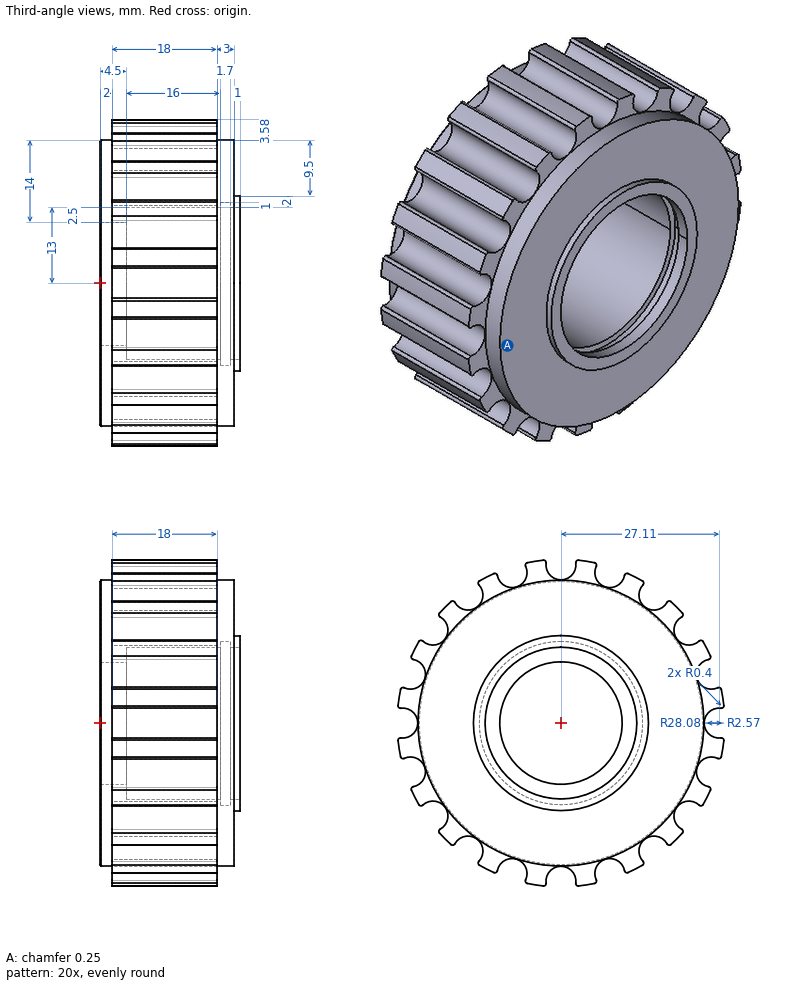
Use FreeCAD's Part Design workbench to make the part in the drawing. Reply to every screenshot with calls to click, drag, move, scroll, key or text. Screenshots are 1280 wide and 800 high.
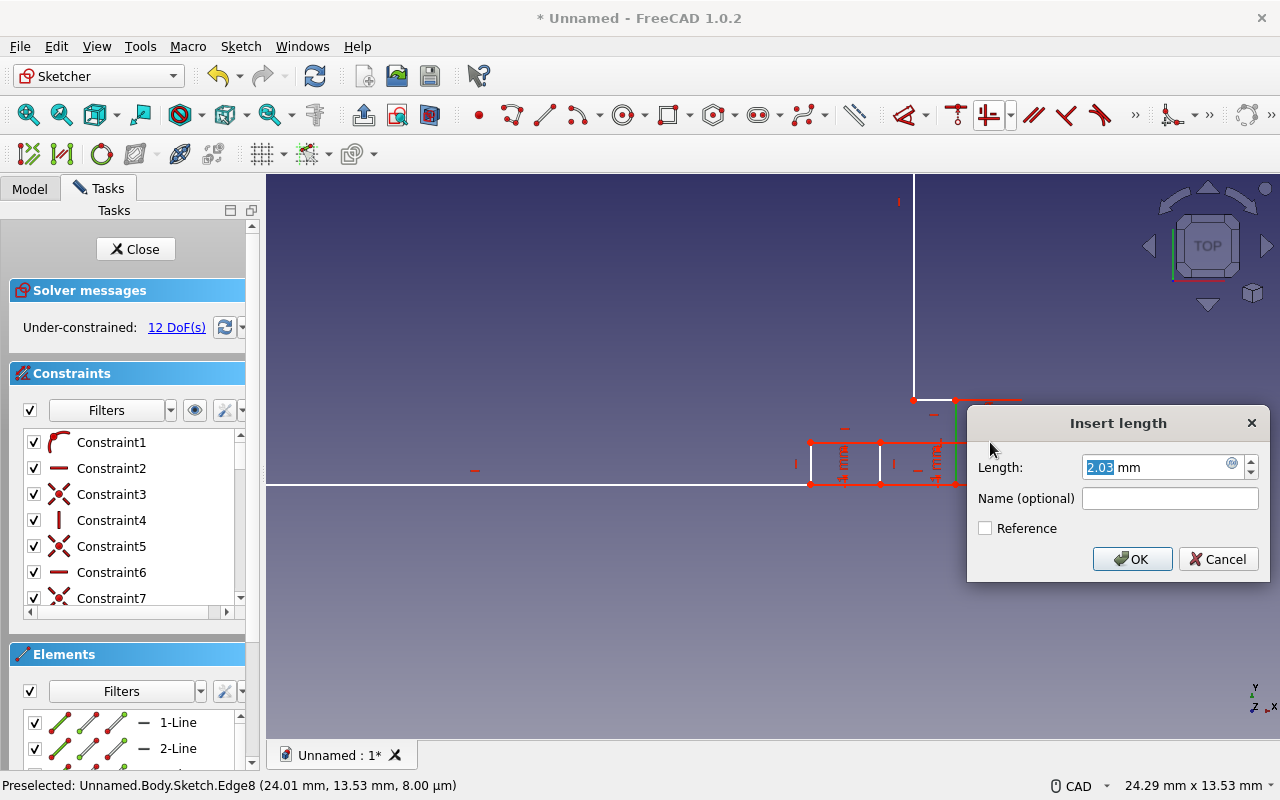
text(2)
key(Return)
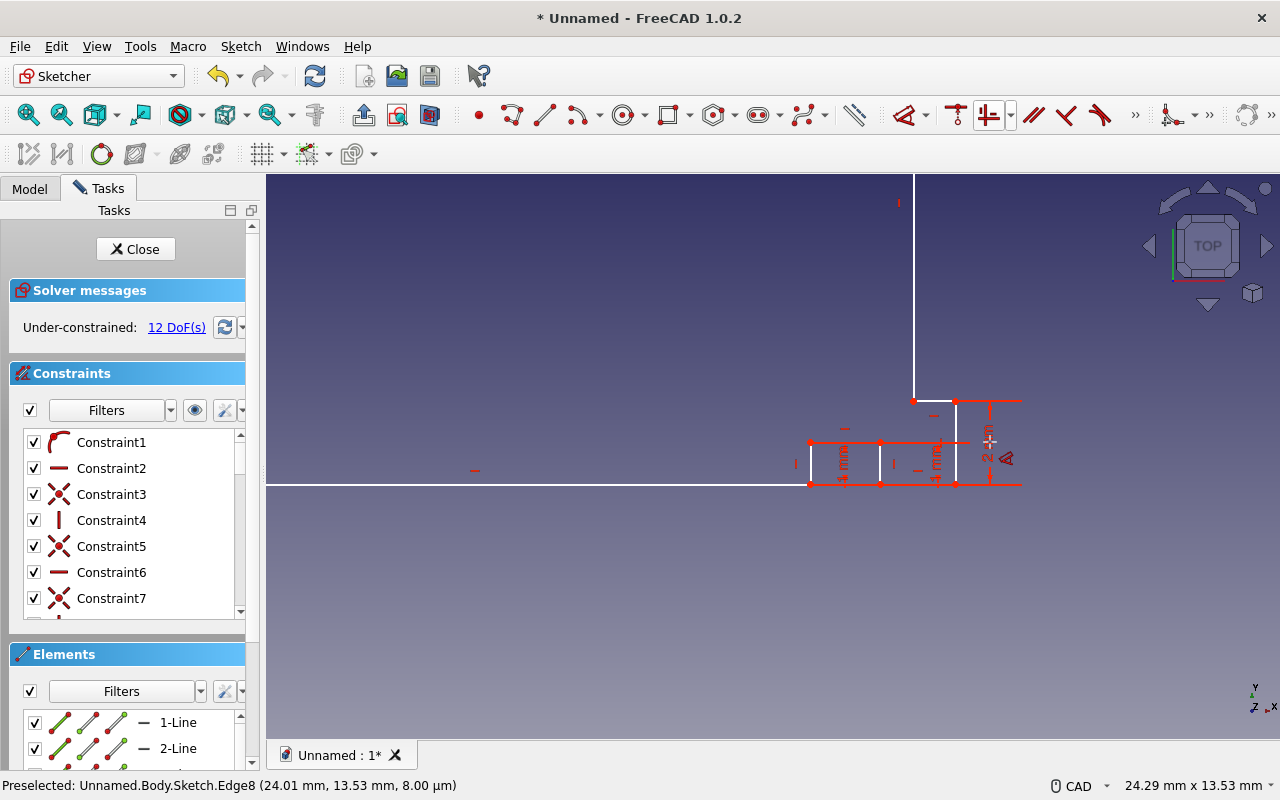
click(943, 401)
click(935, 367)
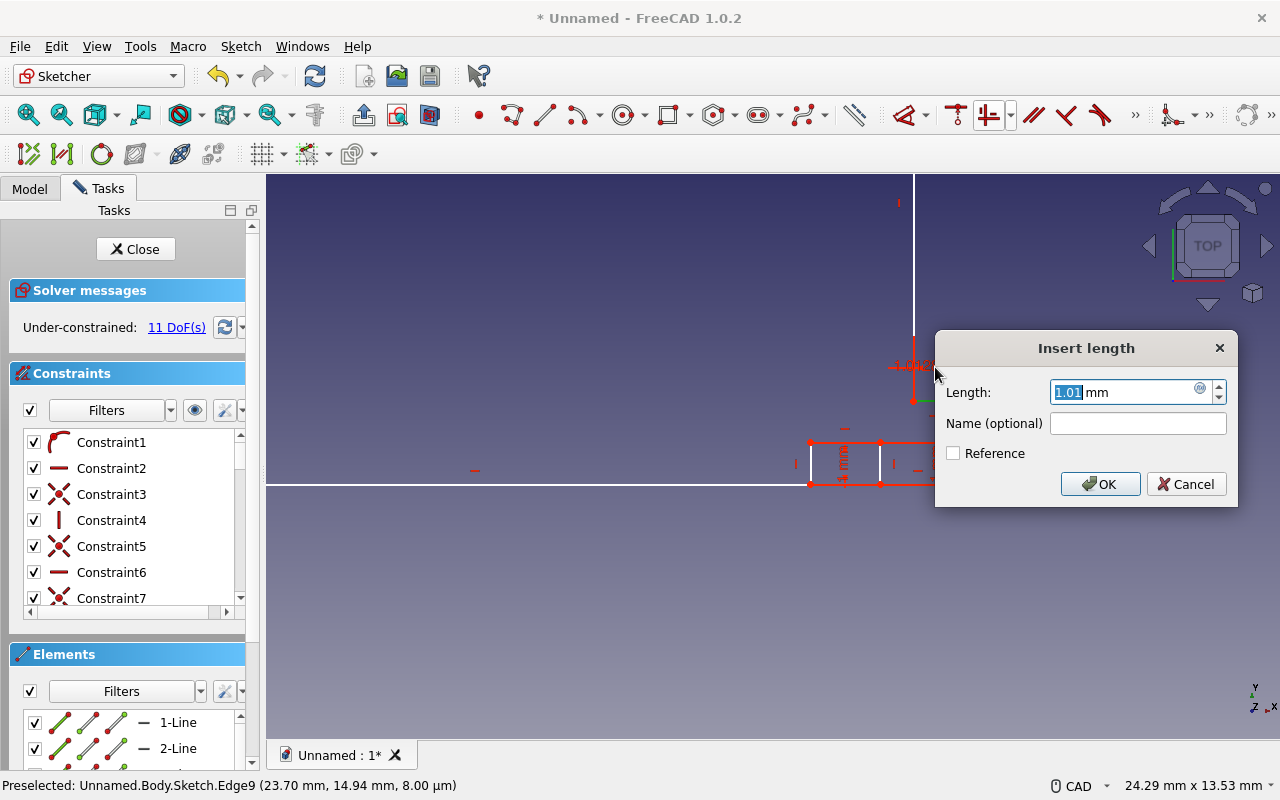
text(1)
key(Return)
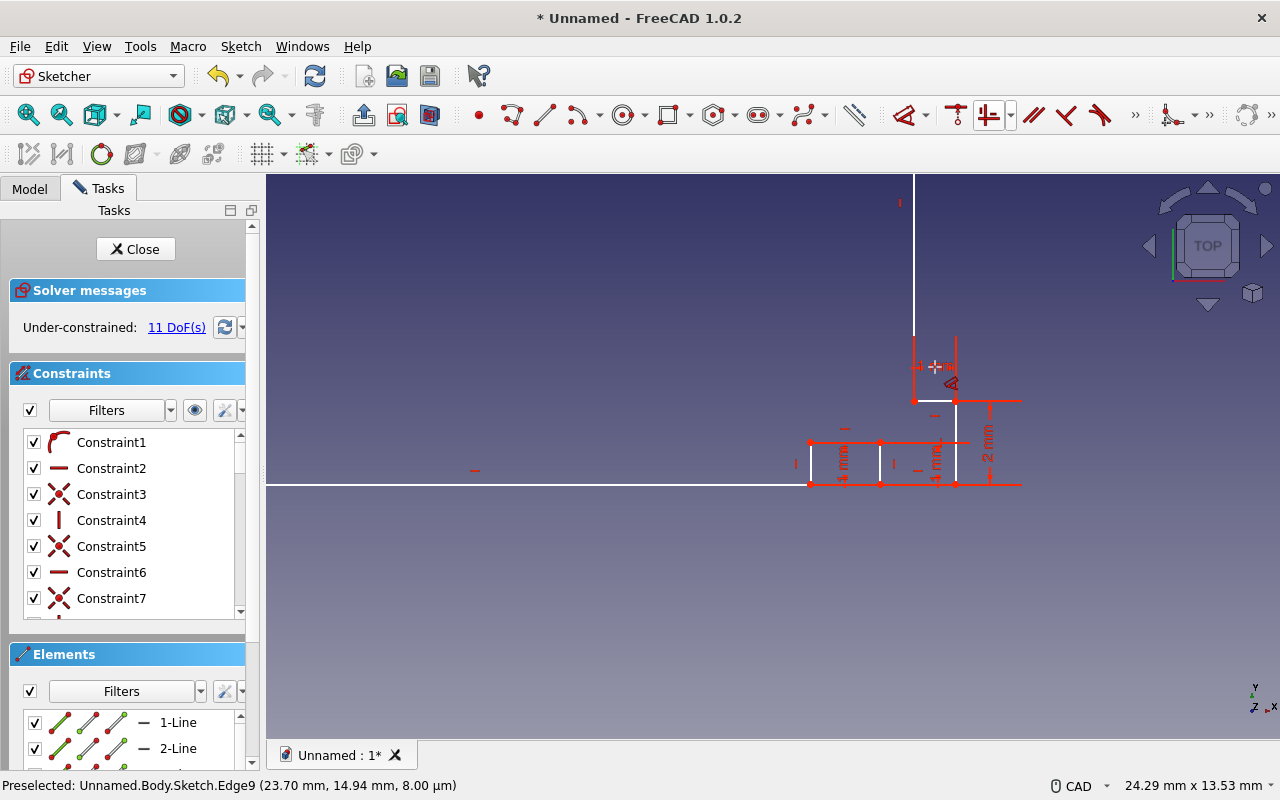
scroll(812, 464, down, 6)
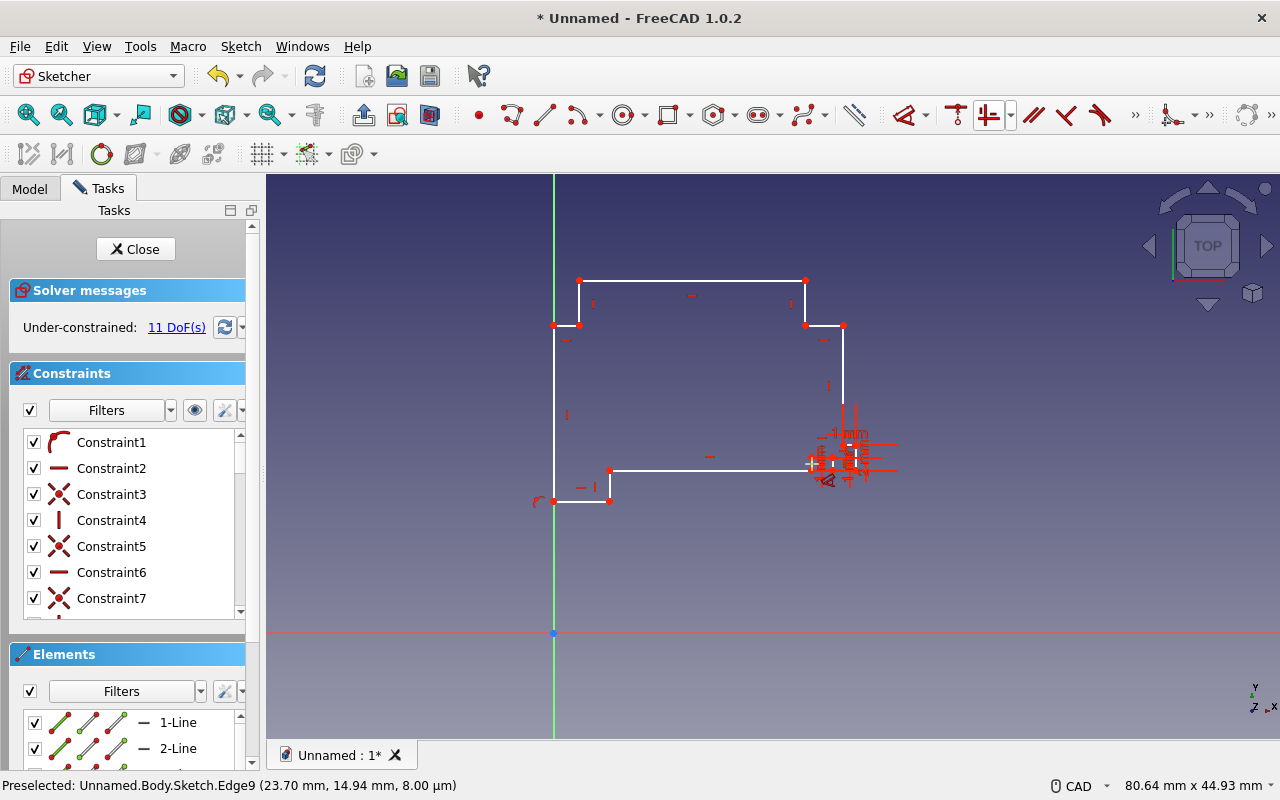
click(832, 326)
click(824, 292)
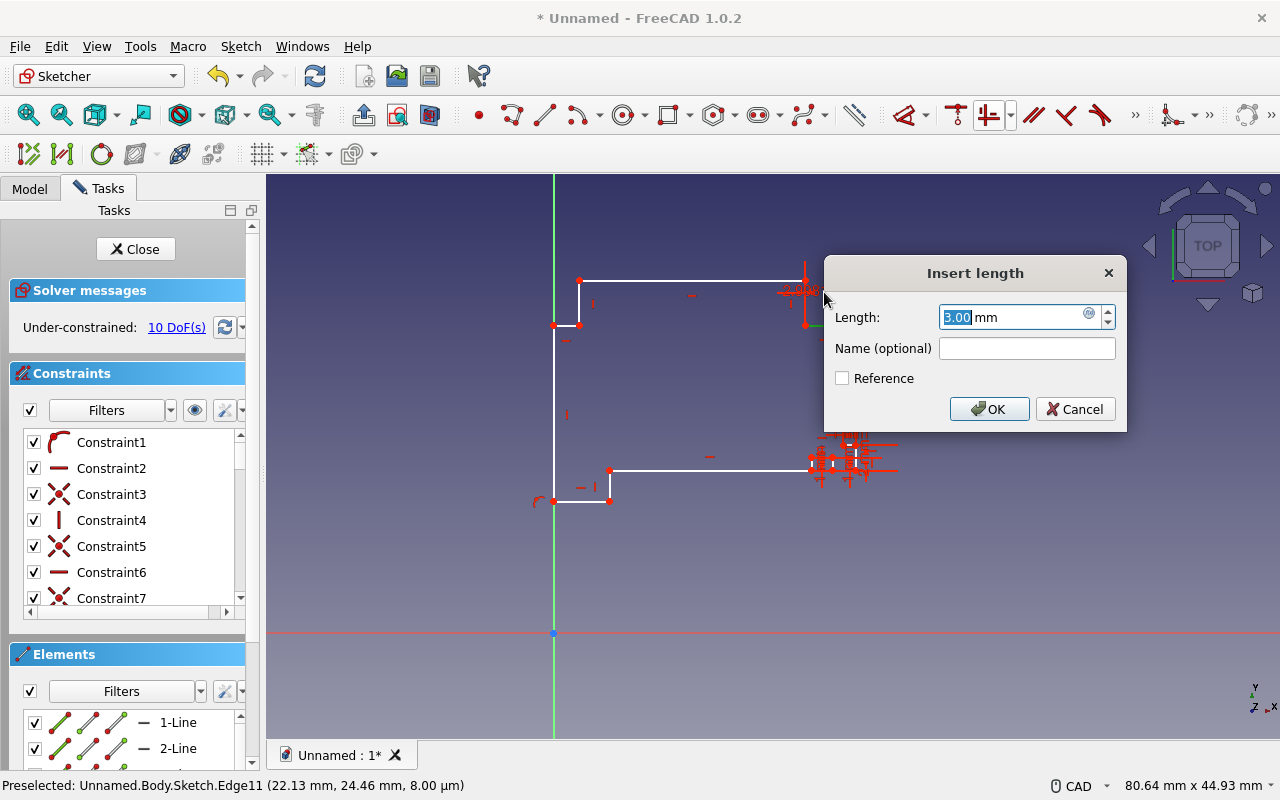
text(3)
key(Return)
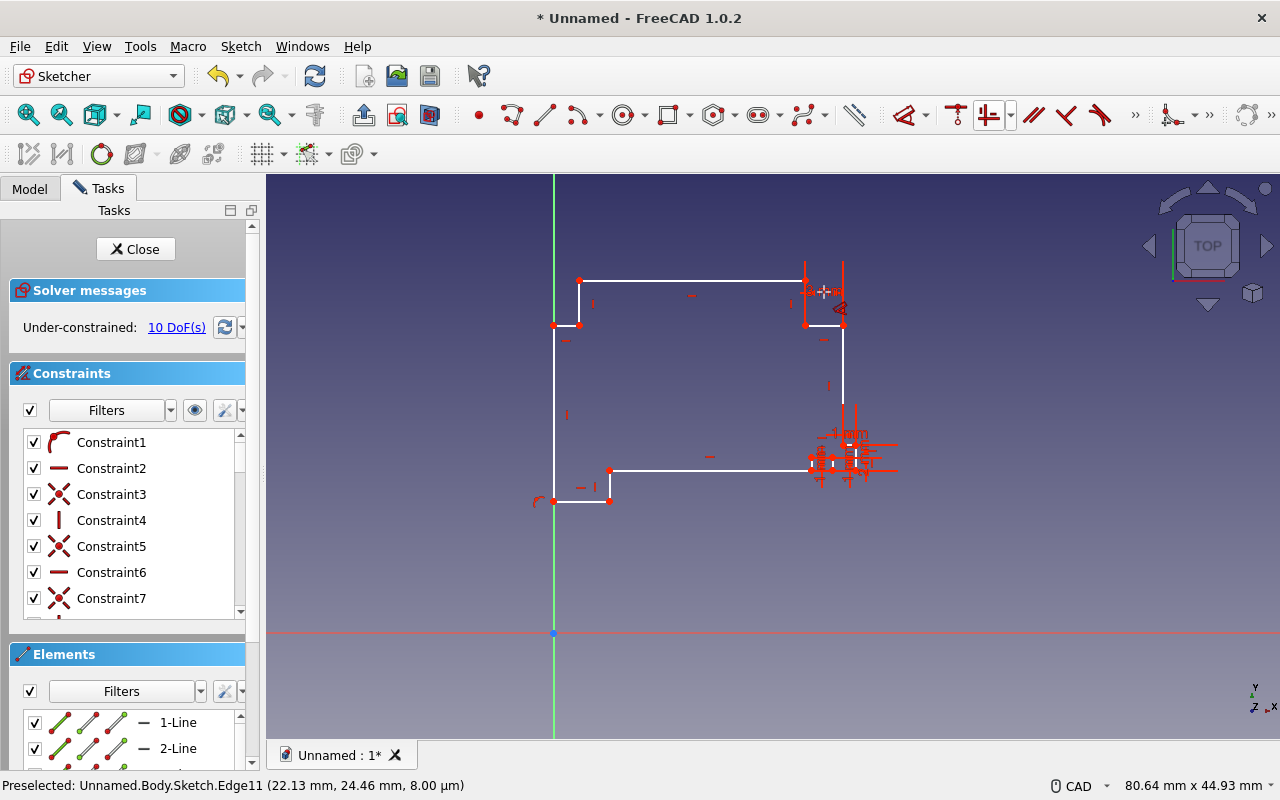
scroll(569, 326, up, 3)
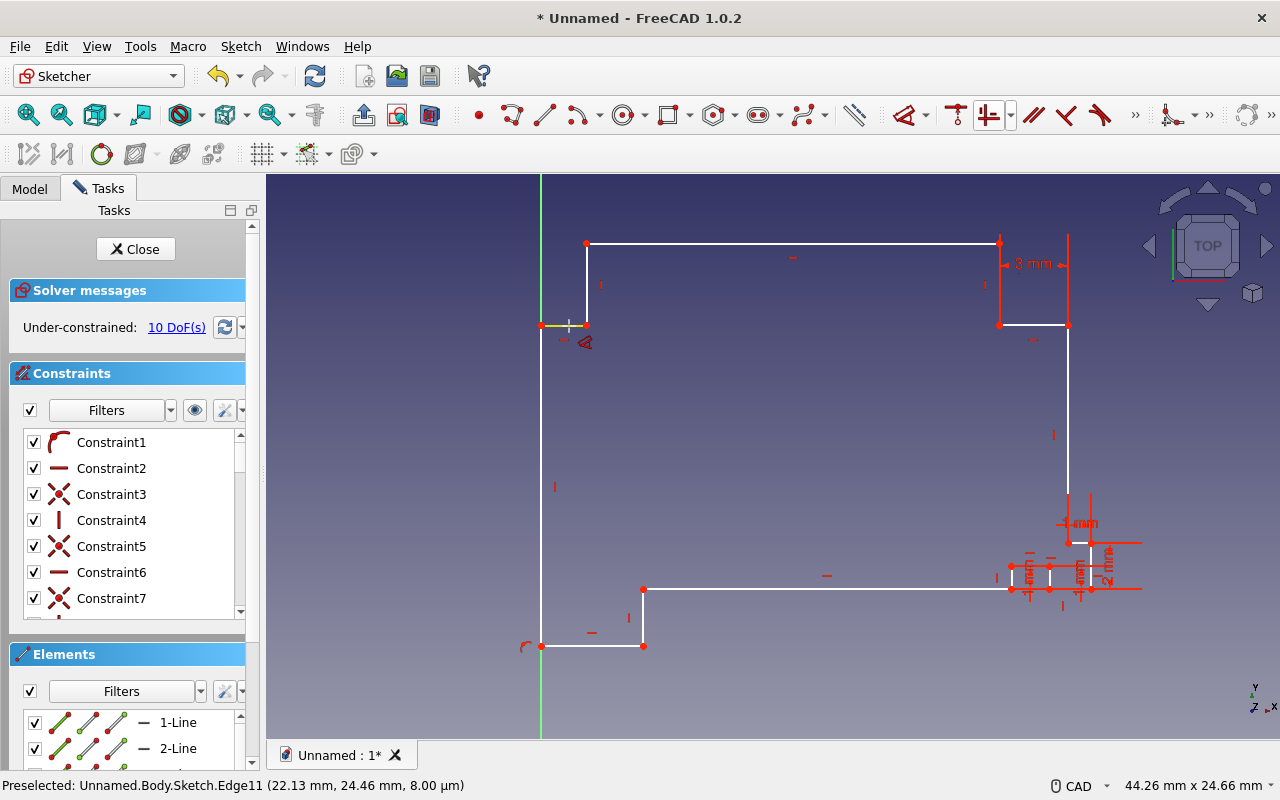
click(569, 326)
click(564, 292)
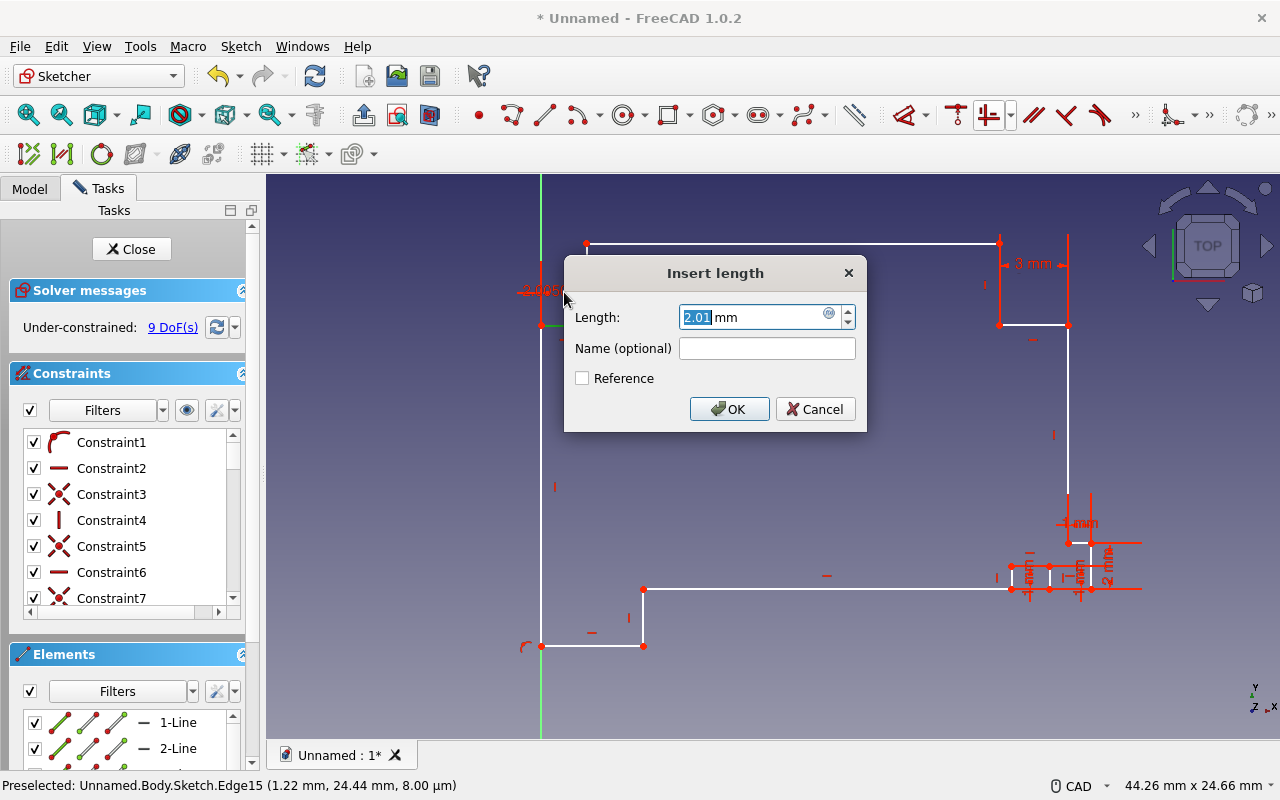
text(2)
key(Return)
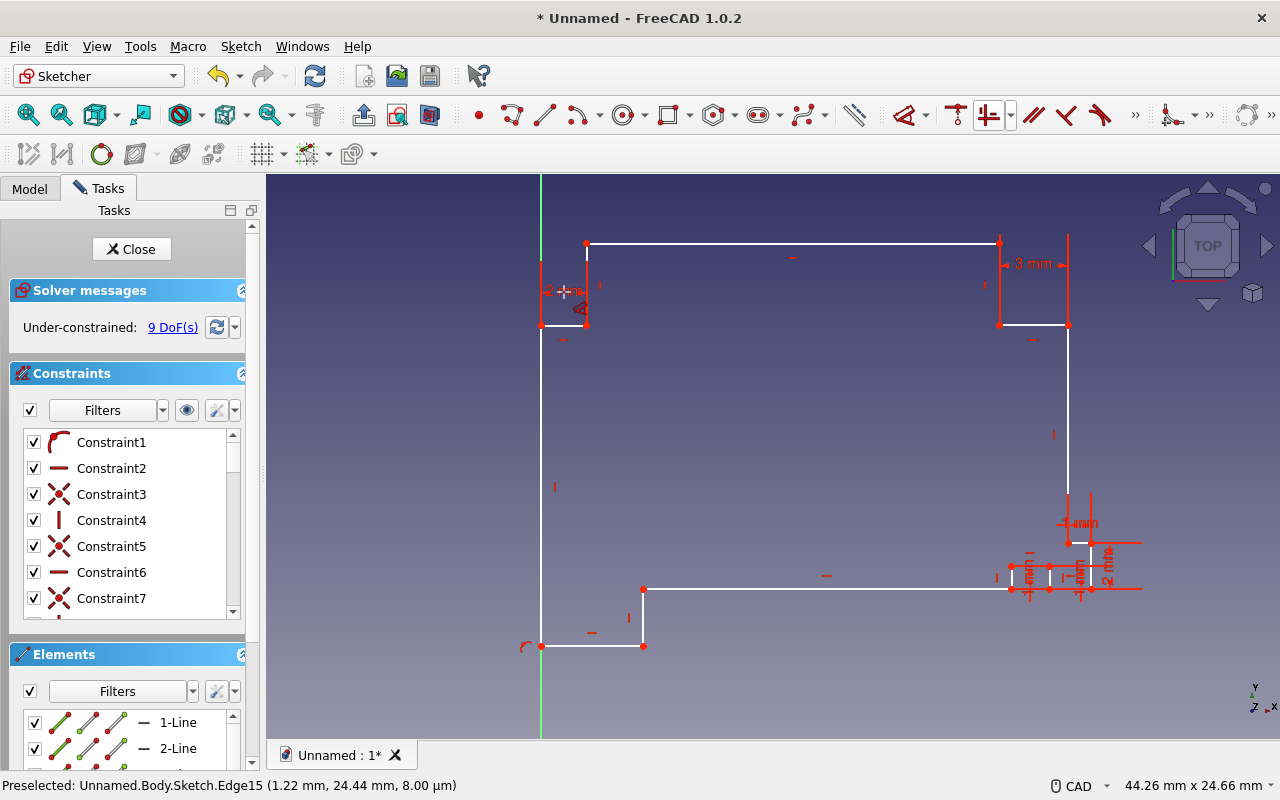
click(754, 589)
click(827, 623)